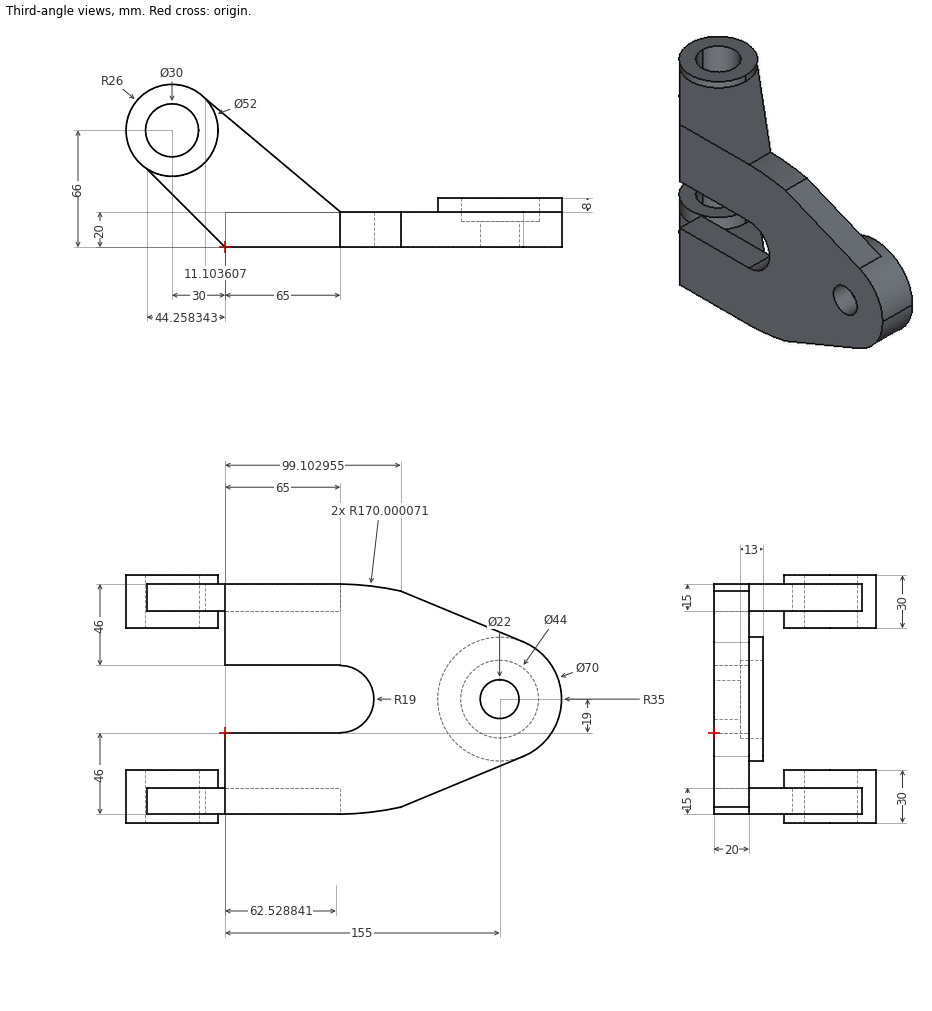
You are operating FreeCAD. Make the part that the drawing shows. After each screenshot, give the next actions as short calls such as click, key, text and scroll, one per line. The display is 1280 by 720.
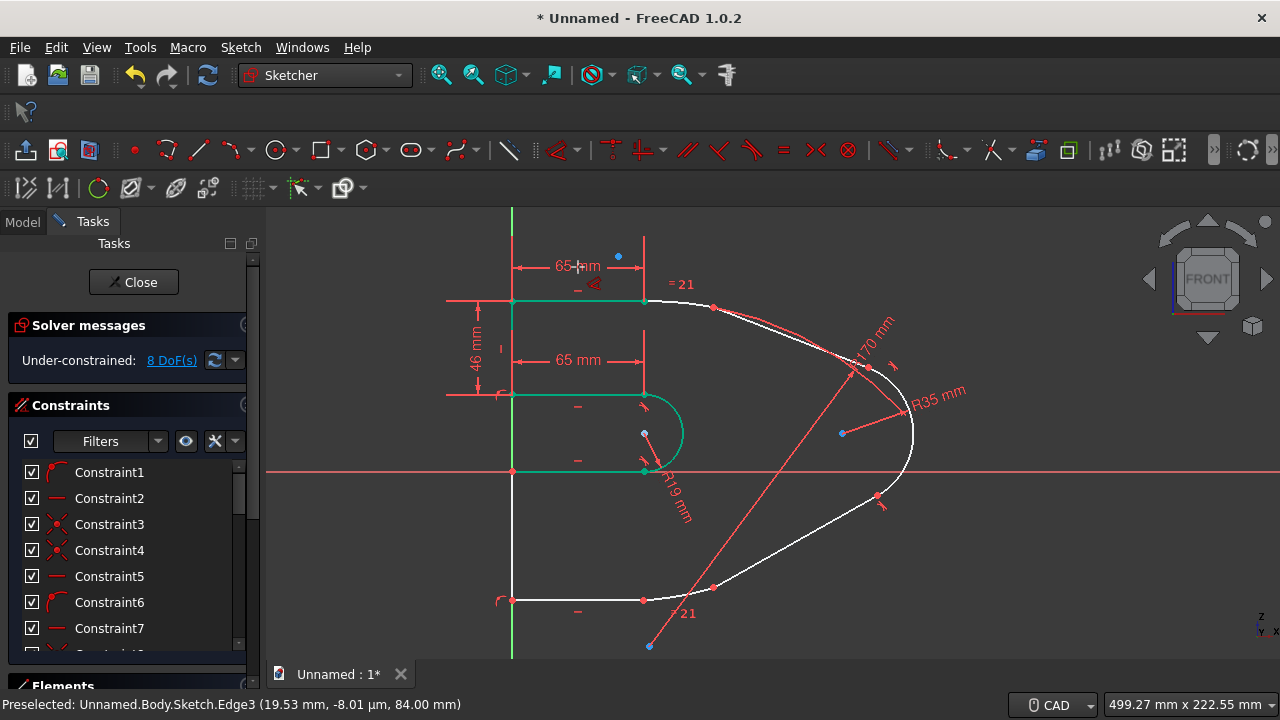
click(604, 600)
click(578, 566)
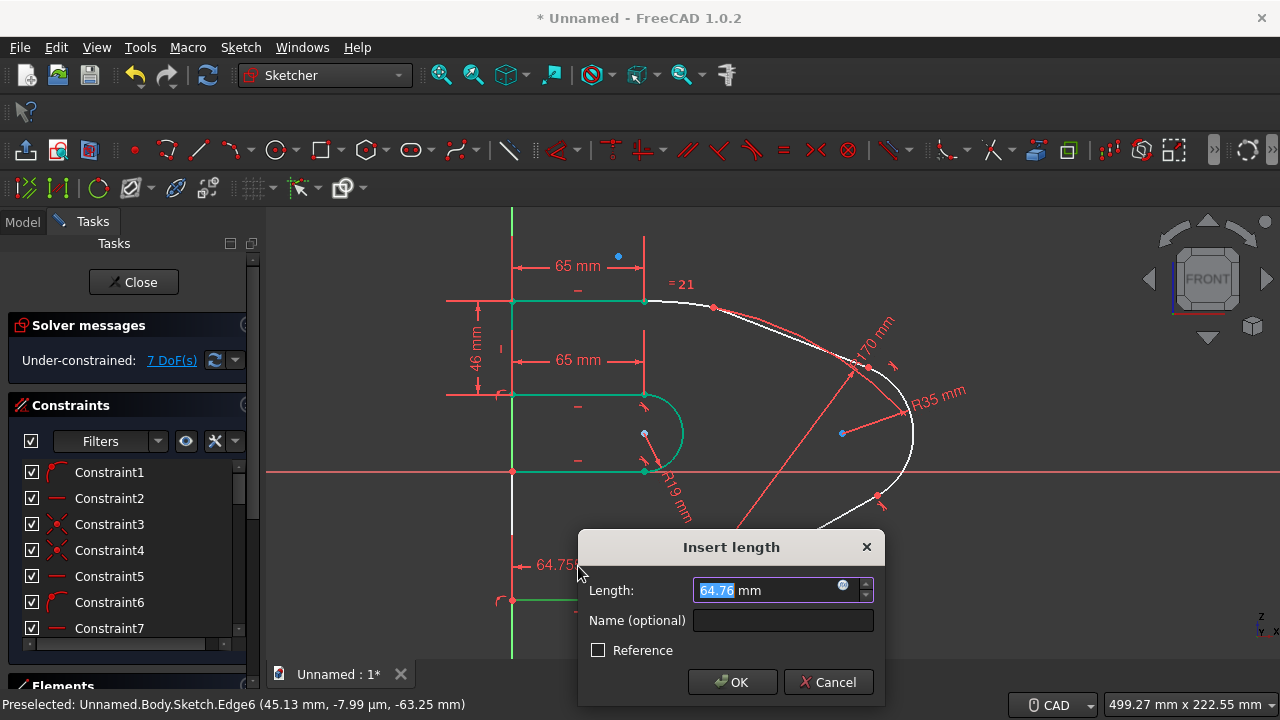
text(65)
key(Return)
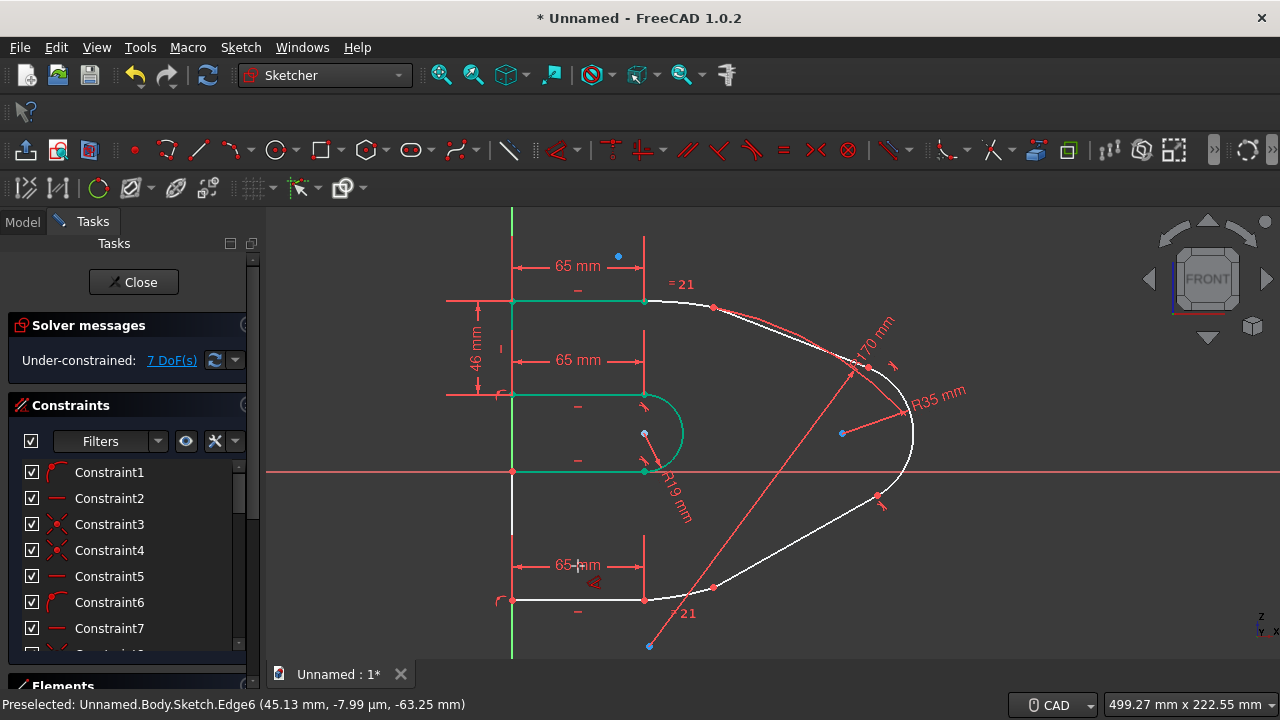
click(512, 562)
click(478, 536)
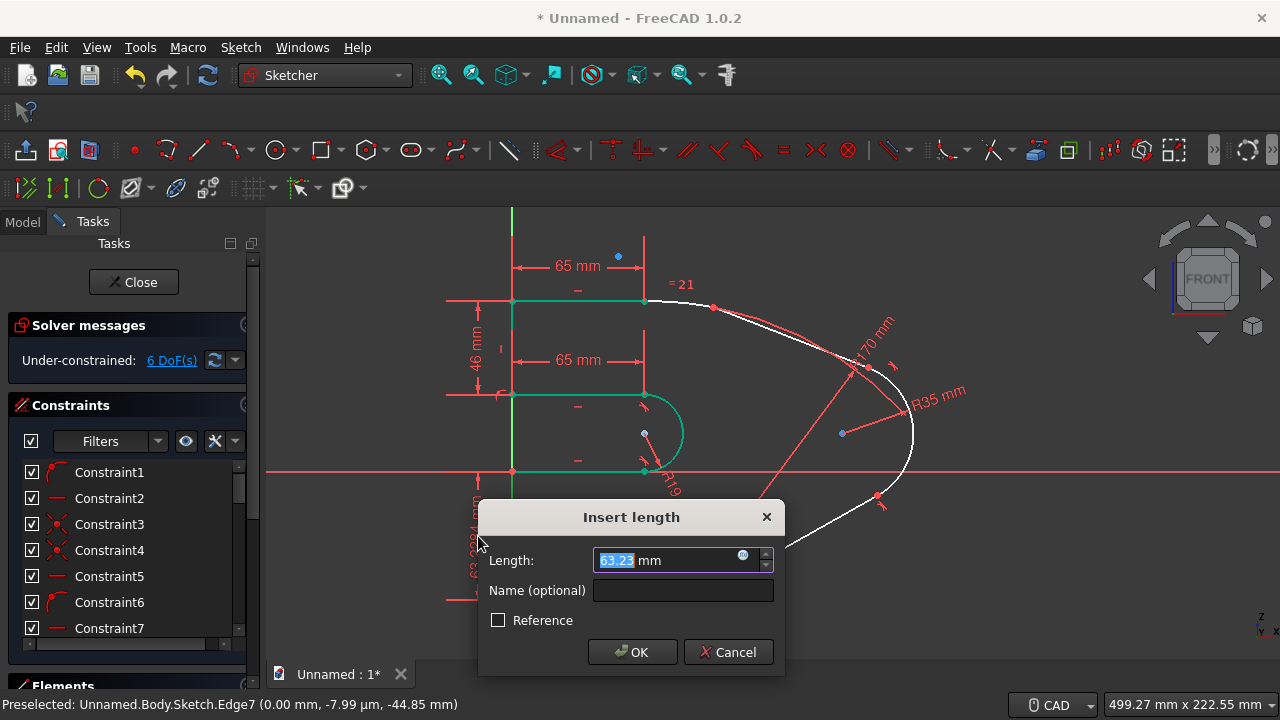
text(46)
key(Return)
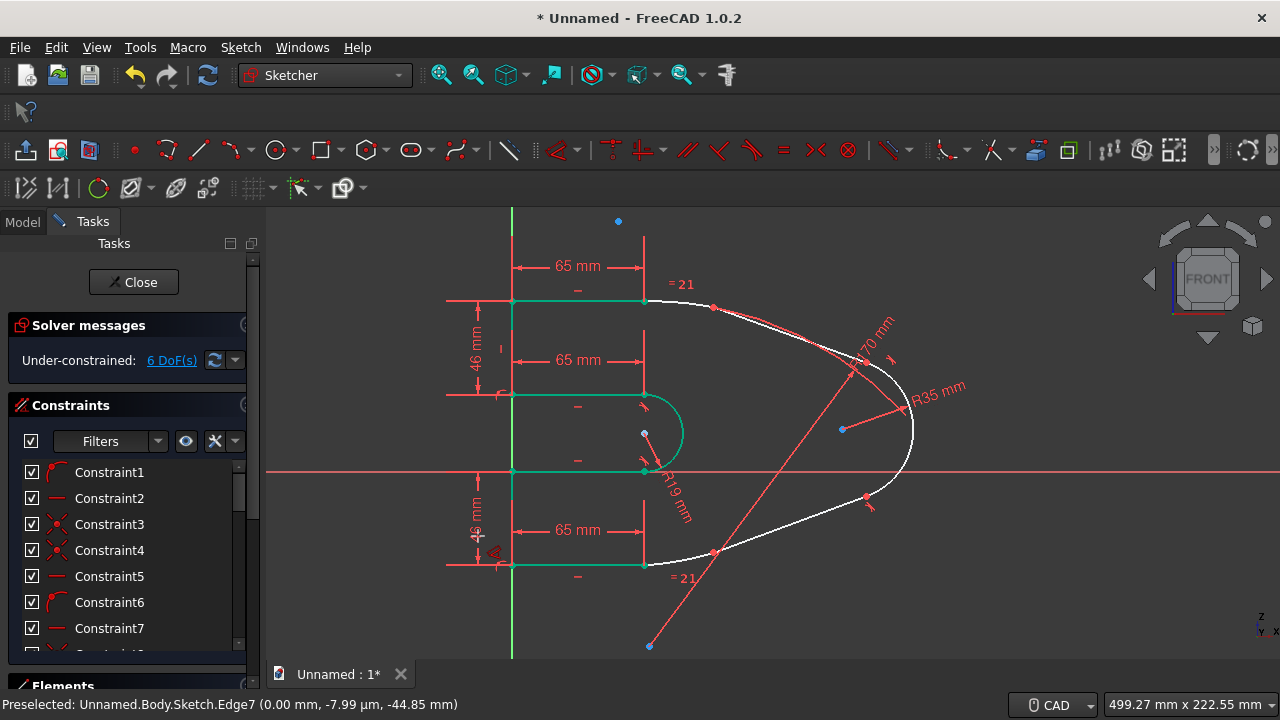
click(842, 430)
click(478, 451)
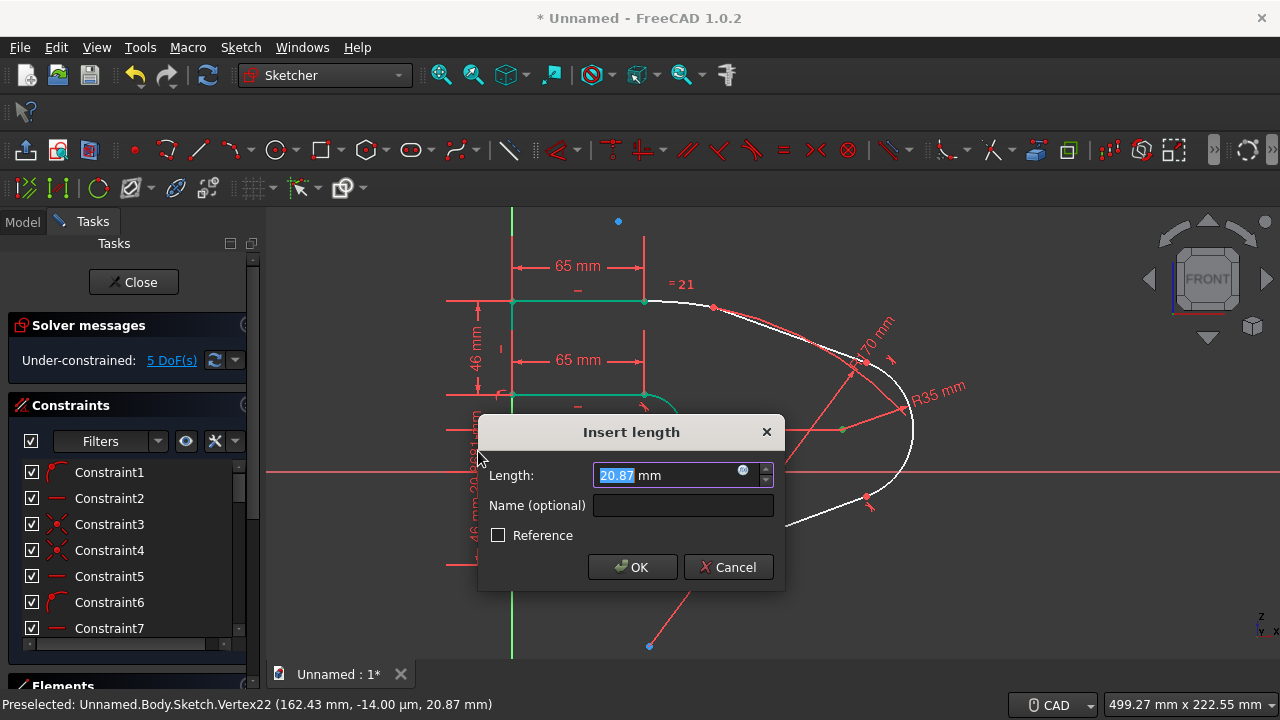
text(19)
key(Return)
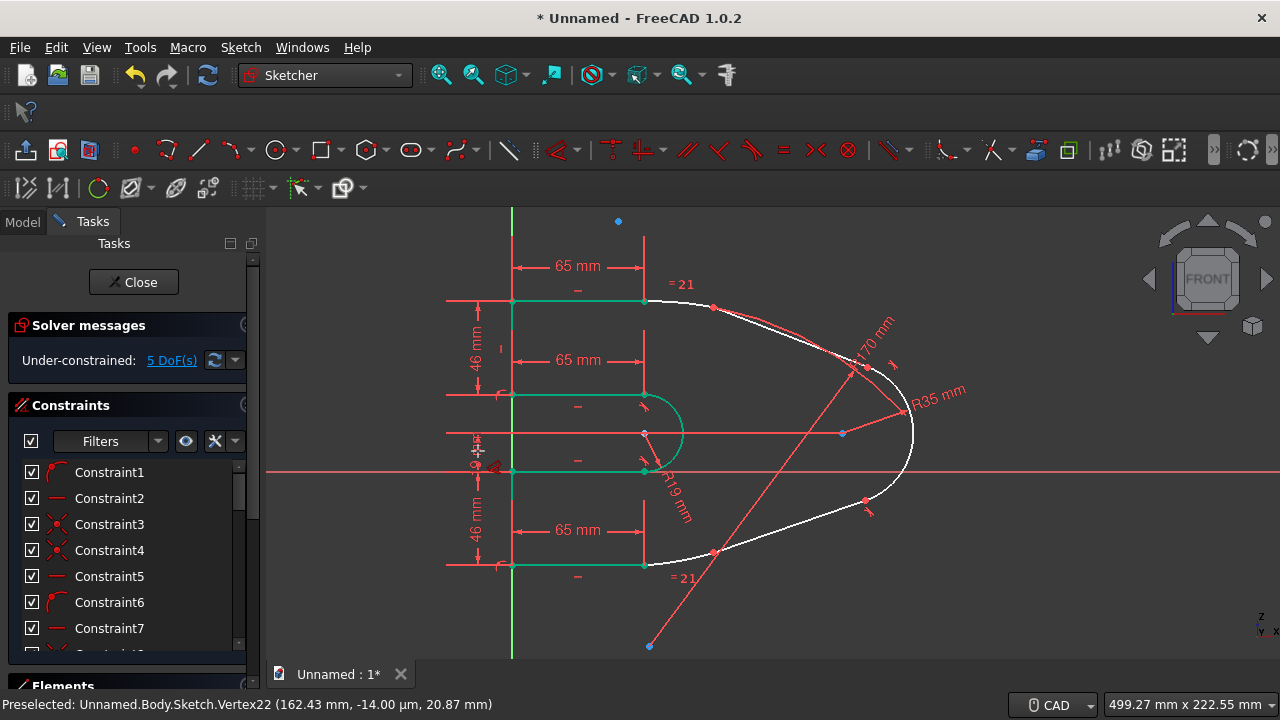
click(842, 433)
click(601, 506)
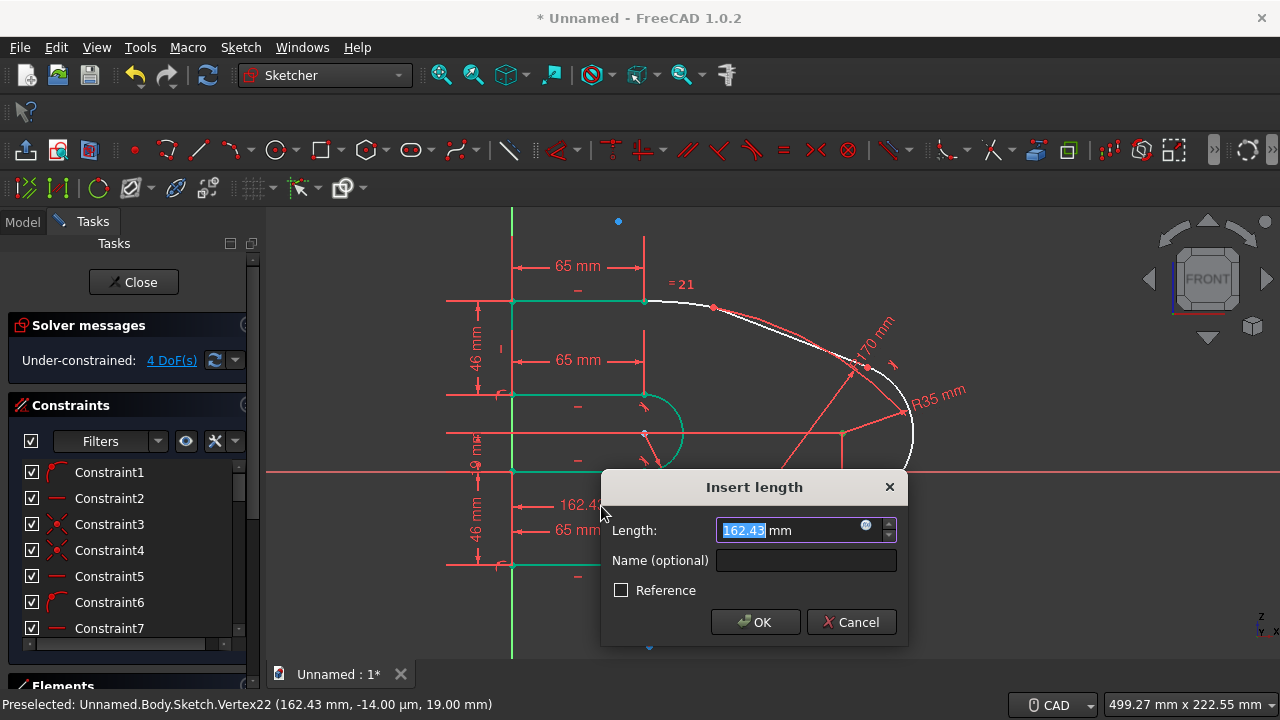
text(155)
key(Return)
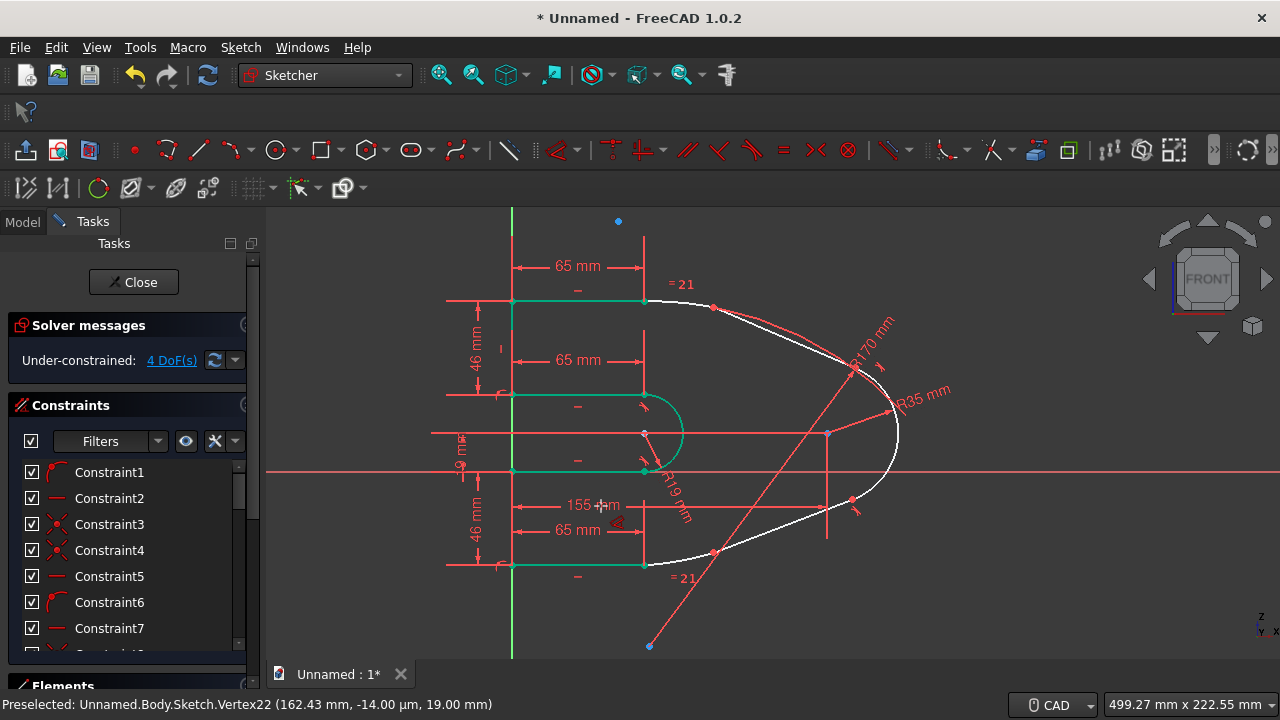
click(714, 307)
click(659, 273)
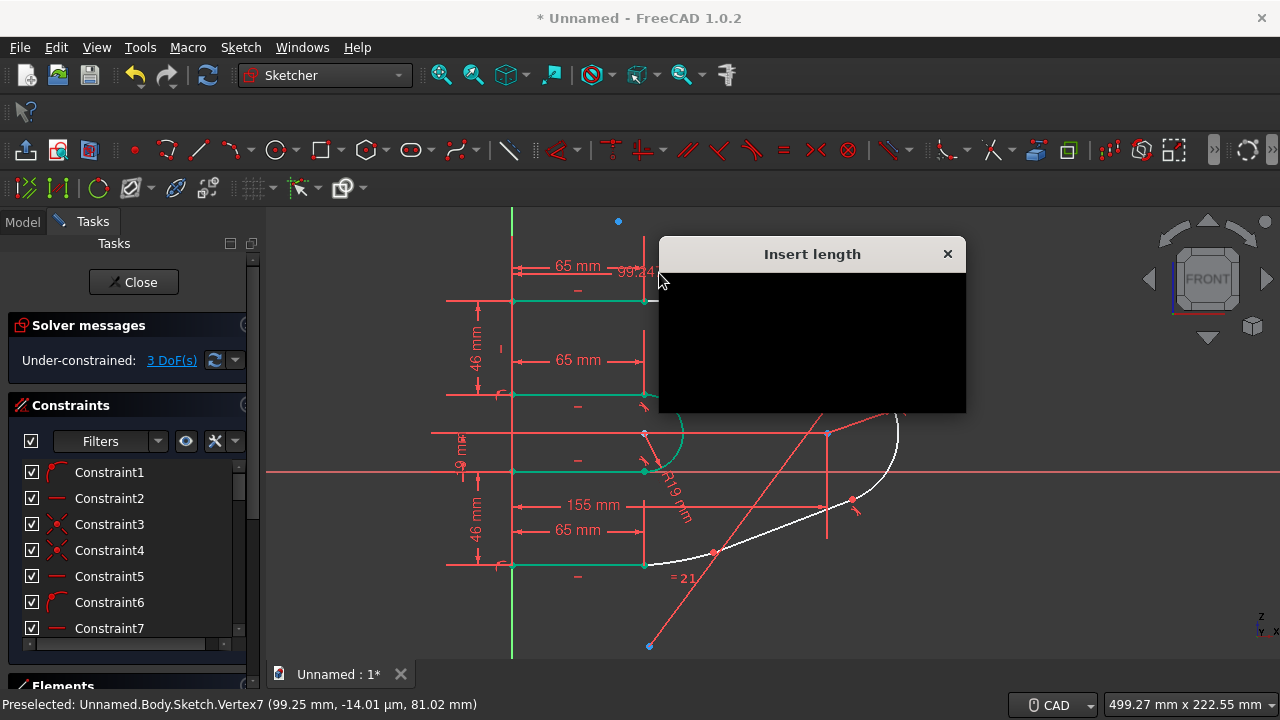
text(99.102955)
key(Return)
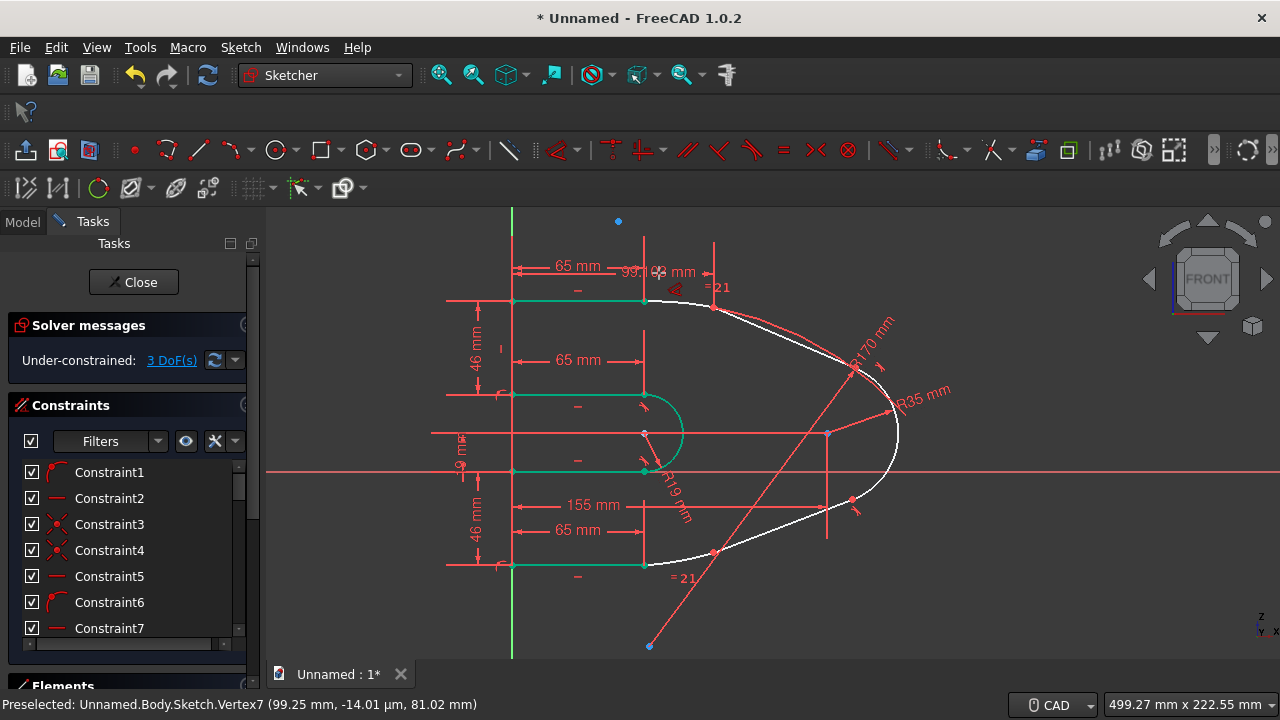
click(714, 553)
click(613, 587)